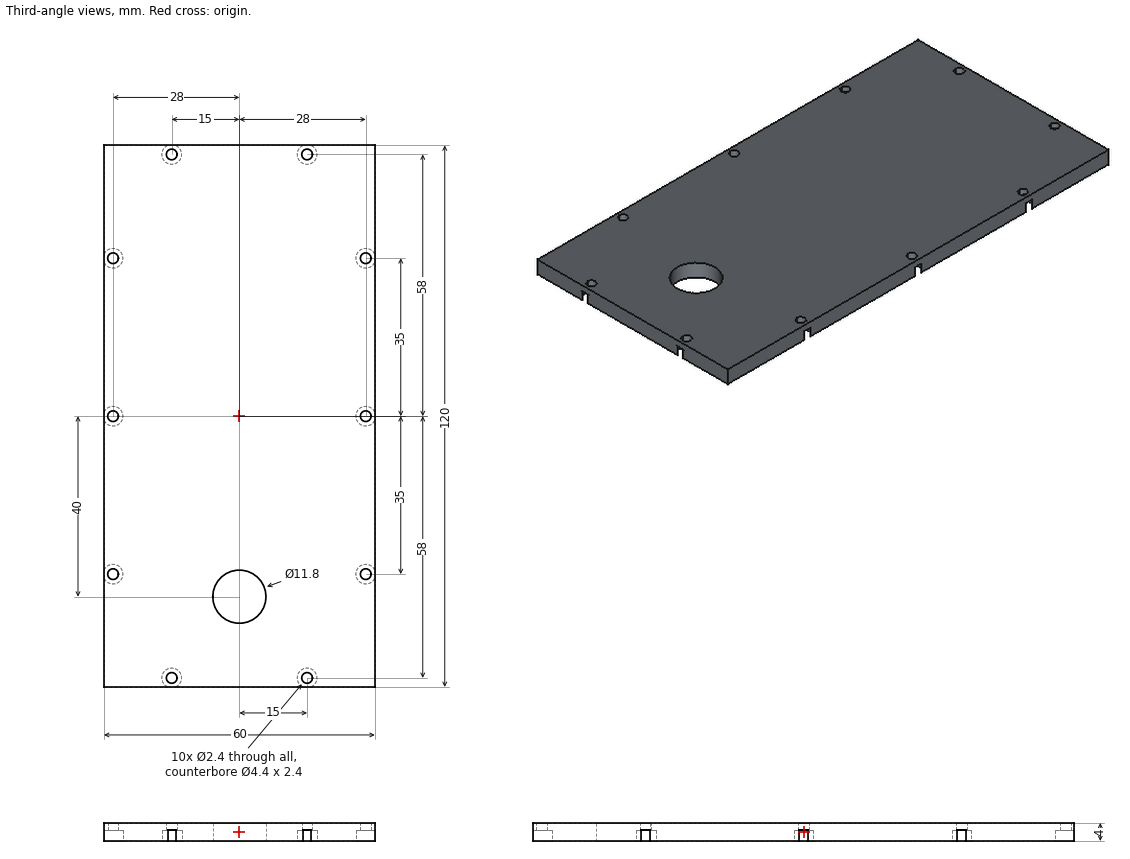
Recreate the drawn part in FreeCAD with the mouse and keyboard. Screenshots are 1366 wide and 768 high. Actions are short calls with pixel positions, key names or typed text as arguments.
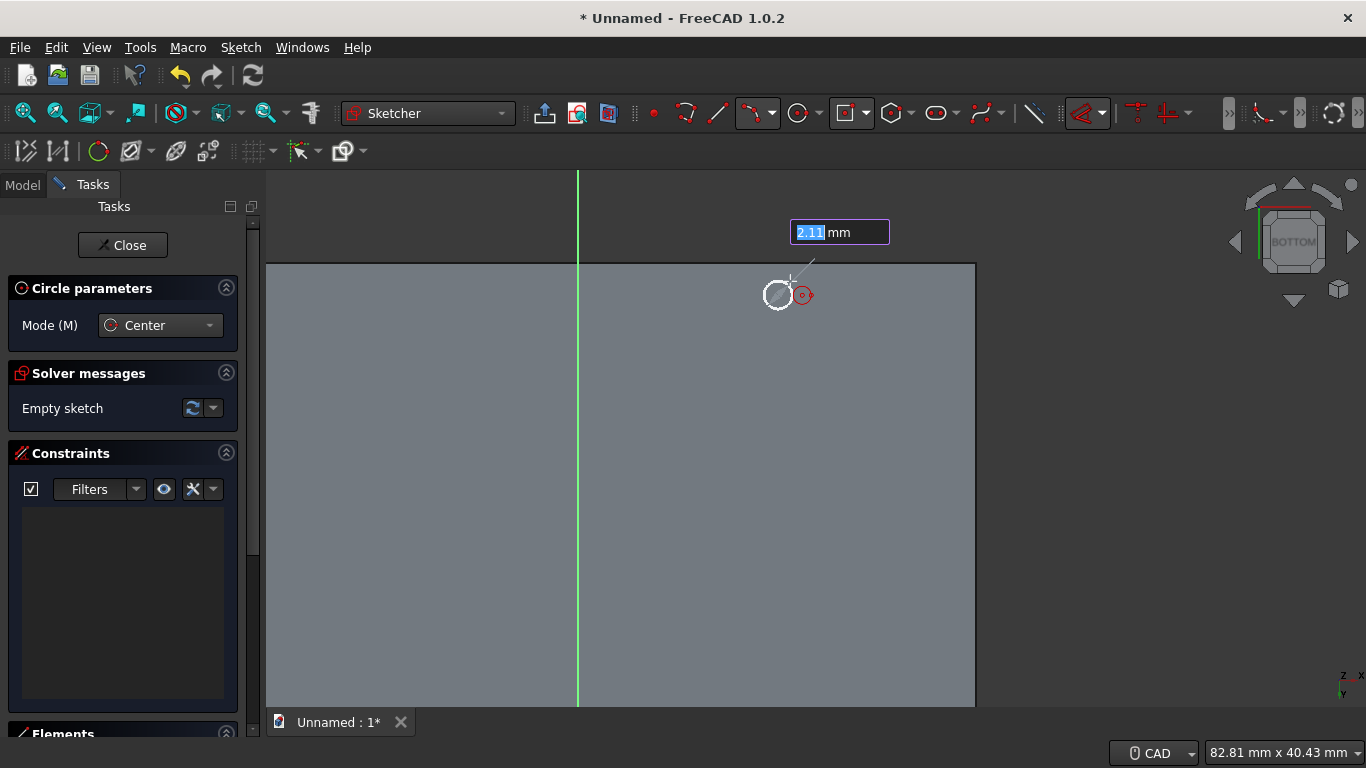
click(788, 279)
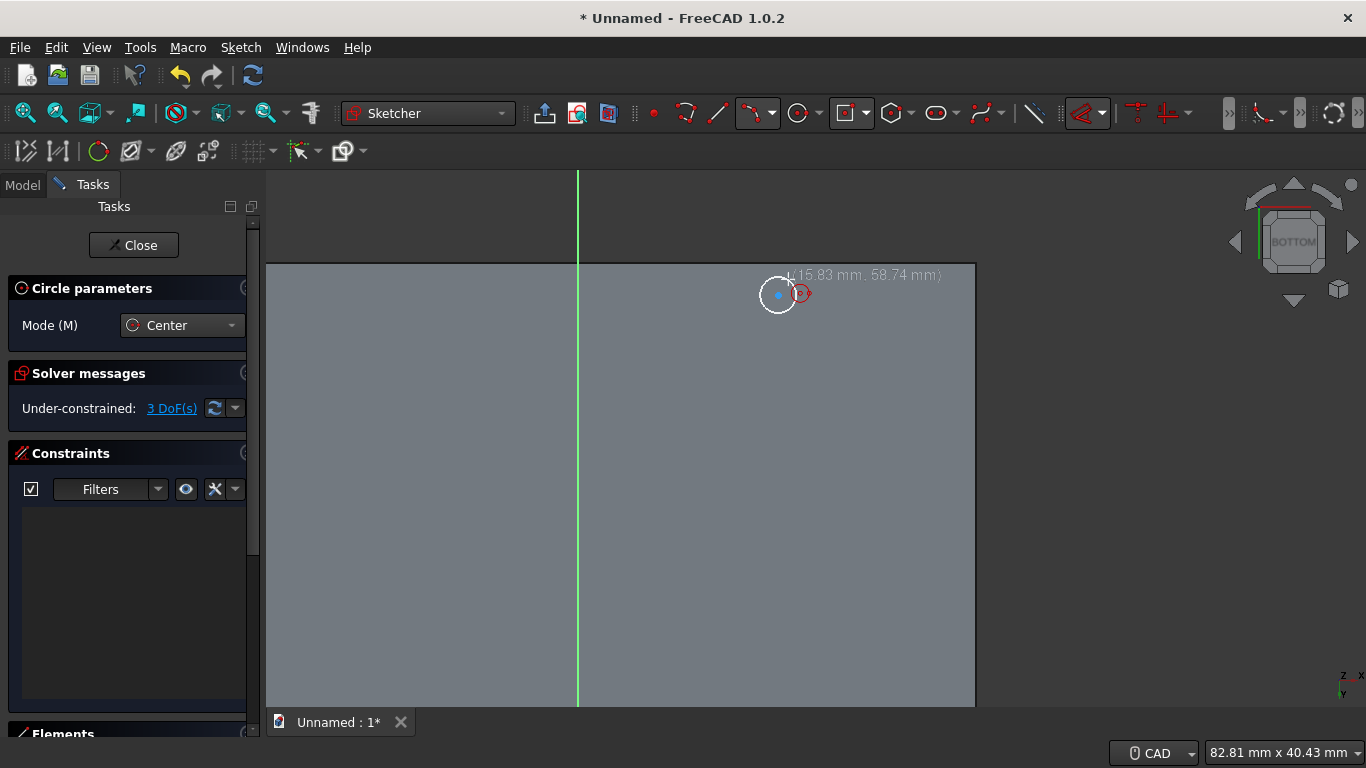
scroll(790, 281, down, 8)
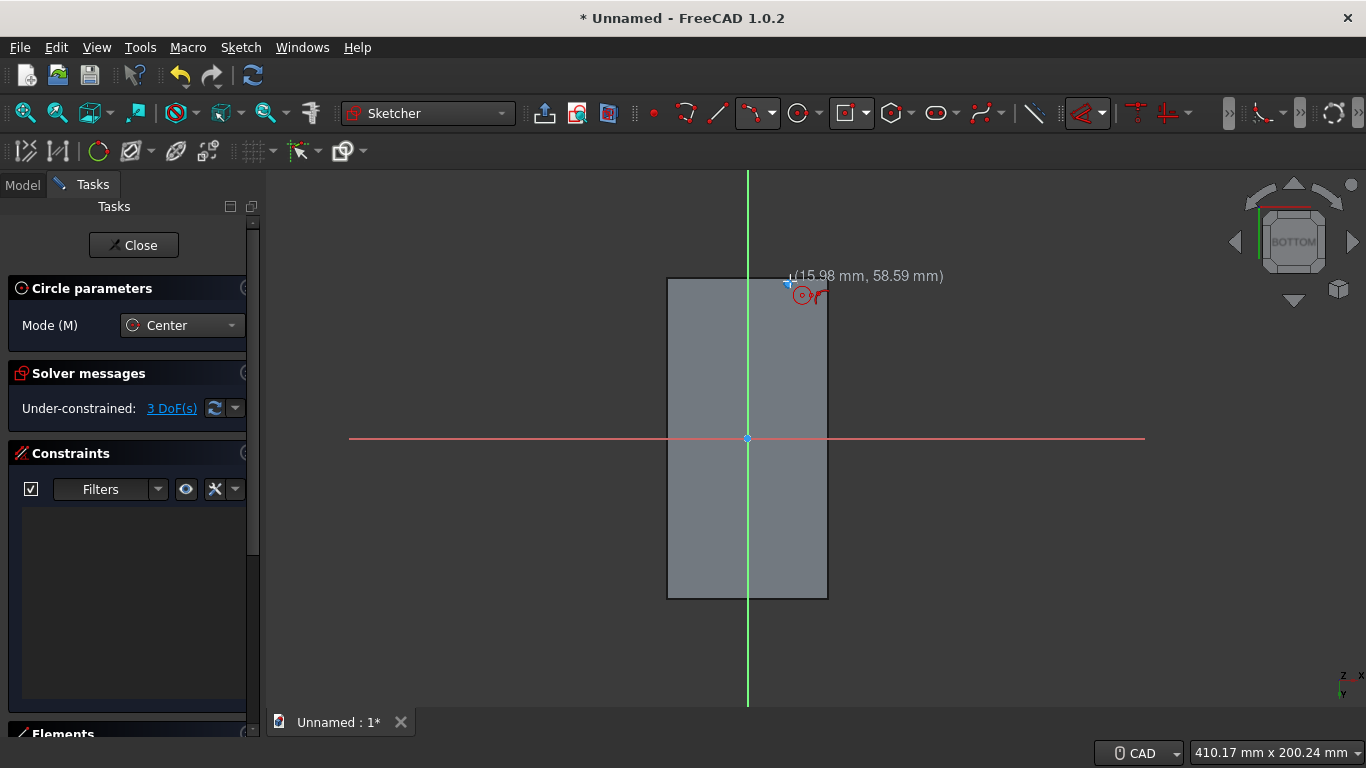
scroll(823, 438, up, 10)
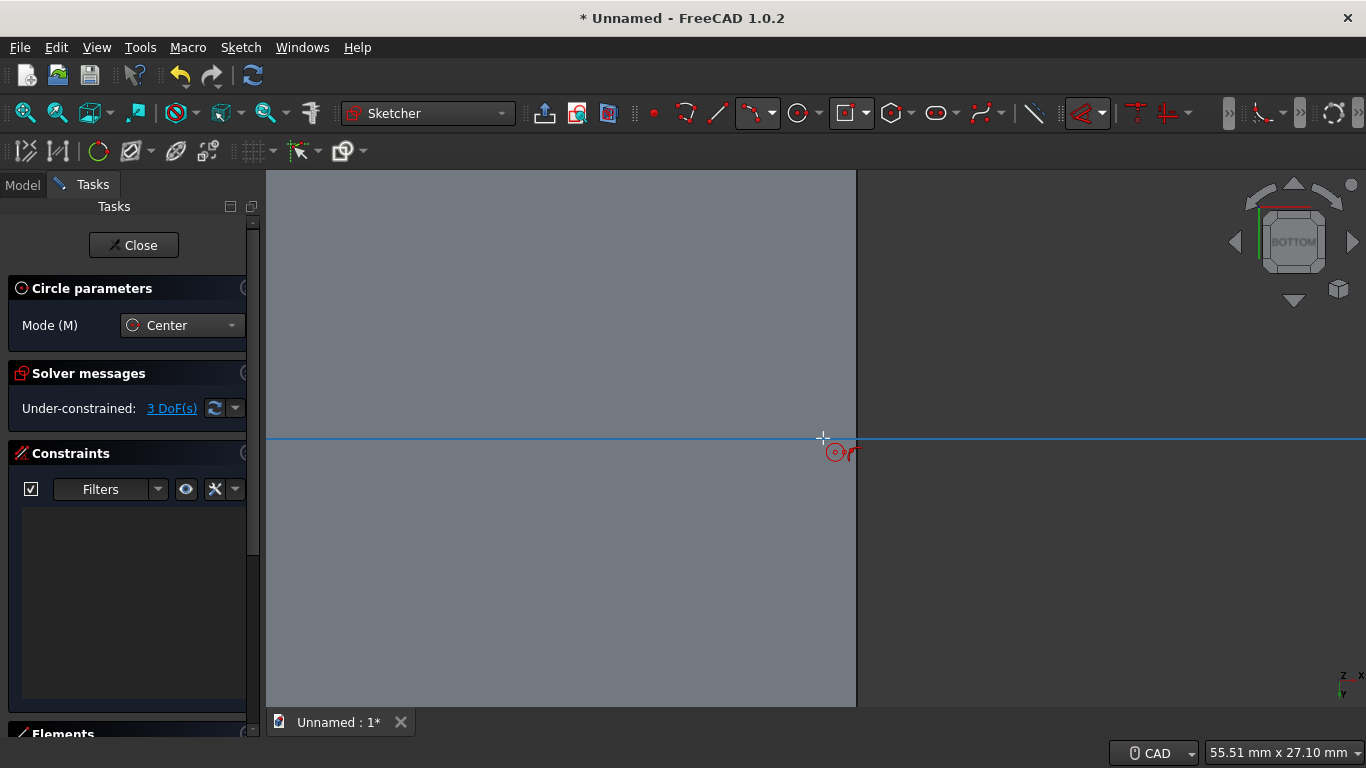
scroll(823, 439, down, 10)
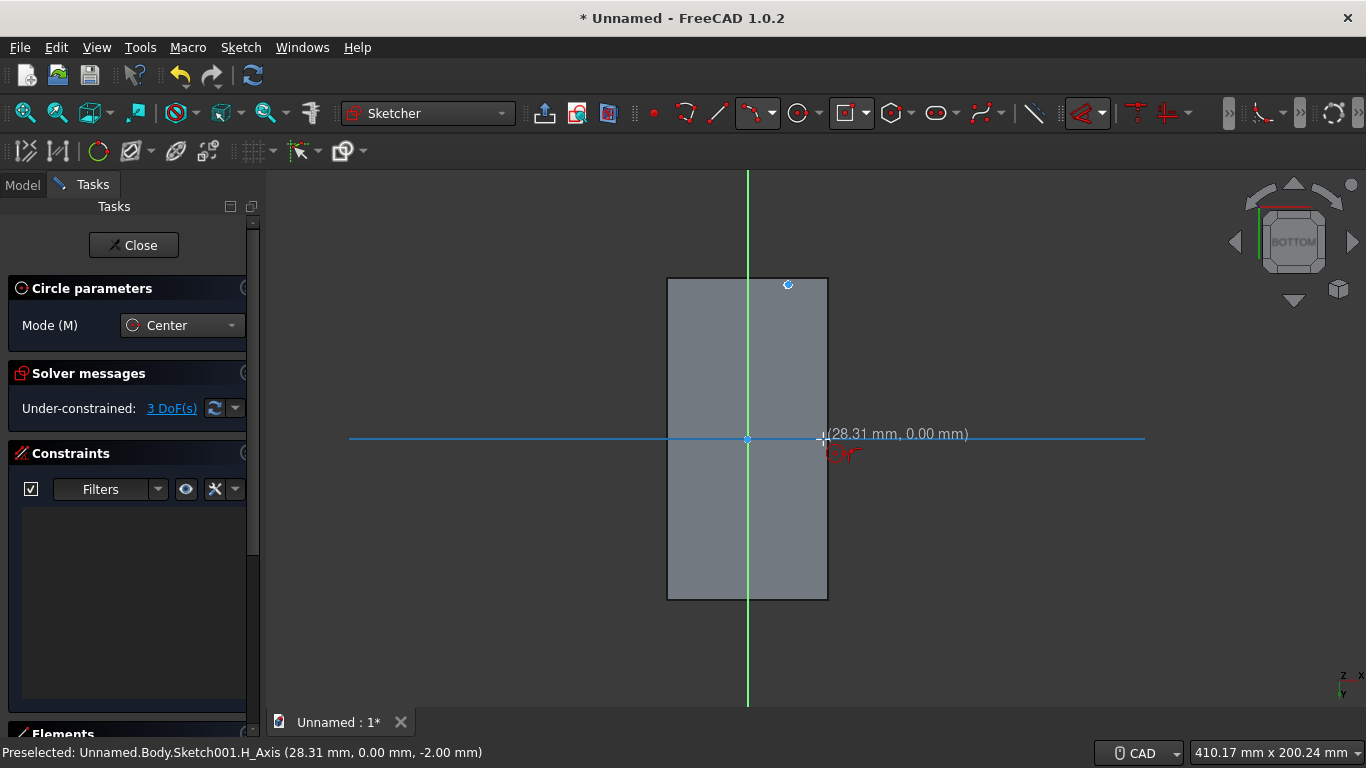
click(823, 439)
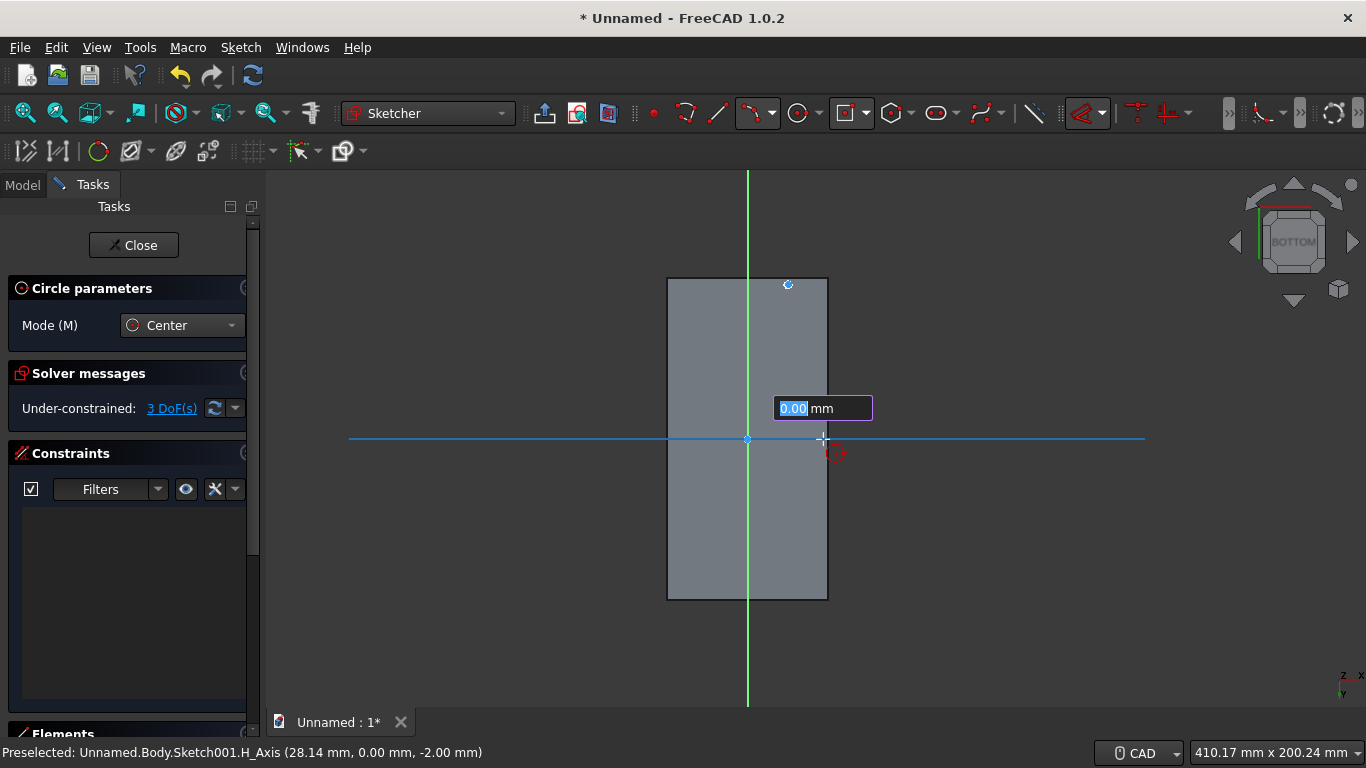
scroll(824, 436, up, 9)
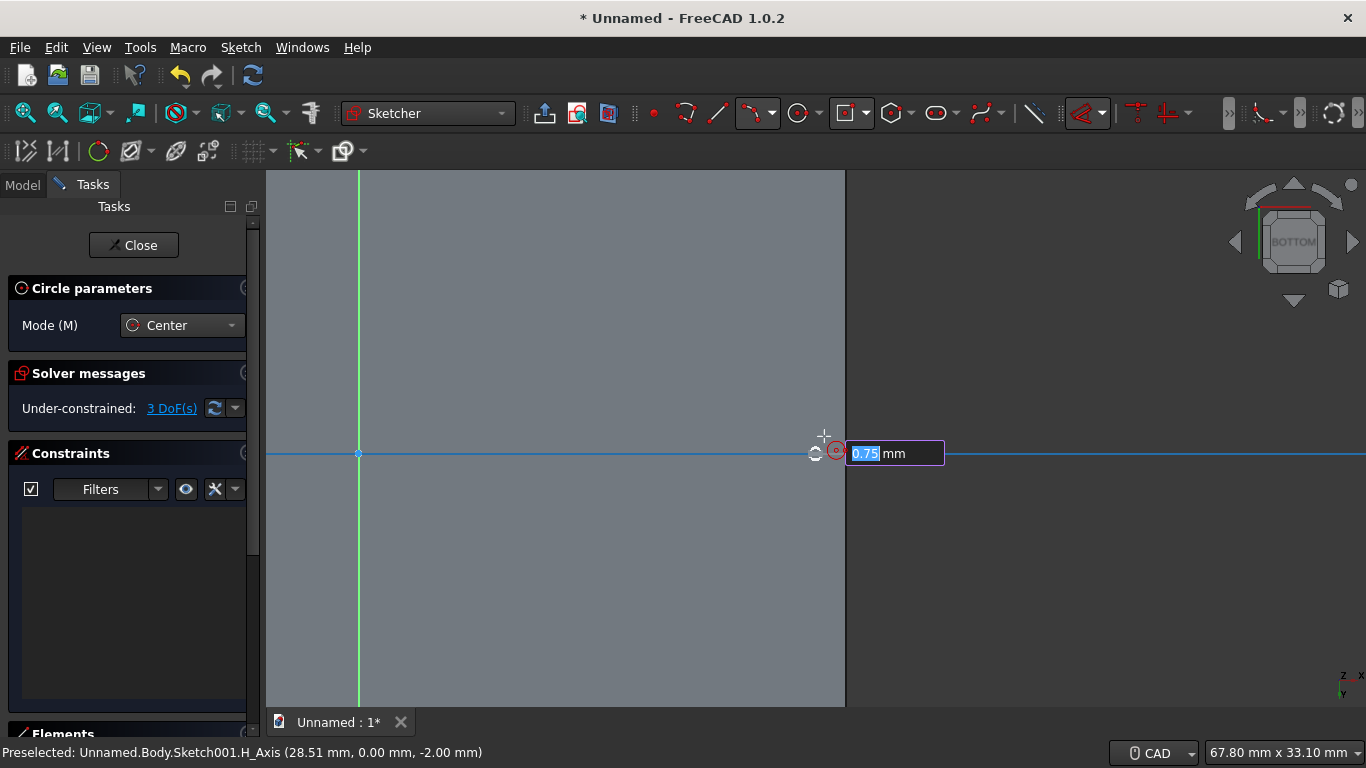
click(820, 436)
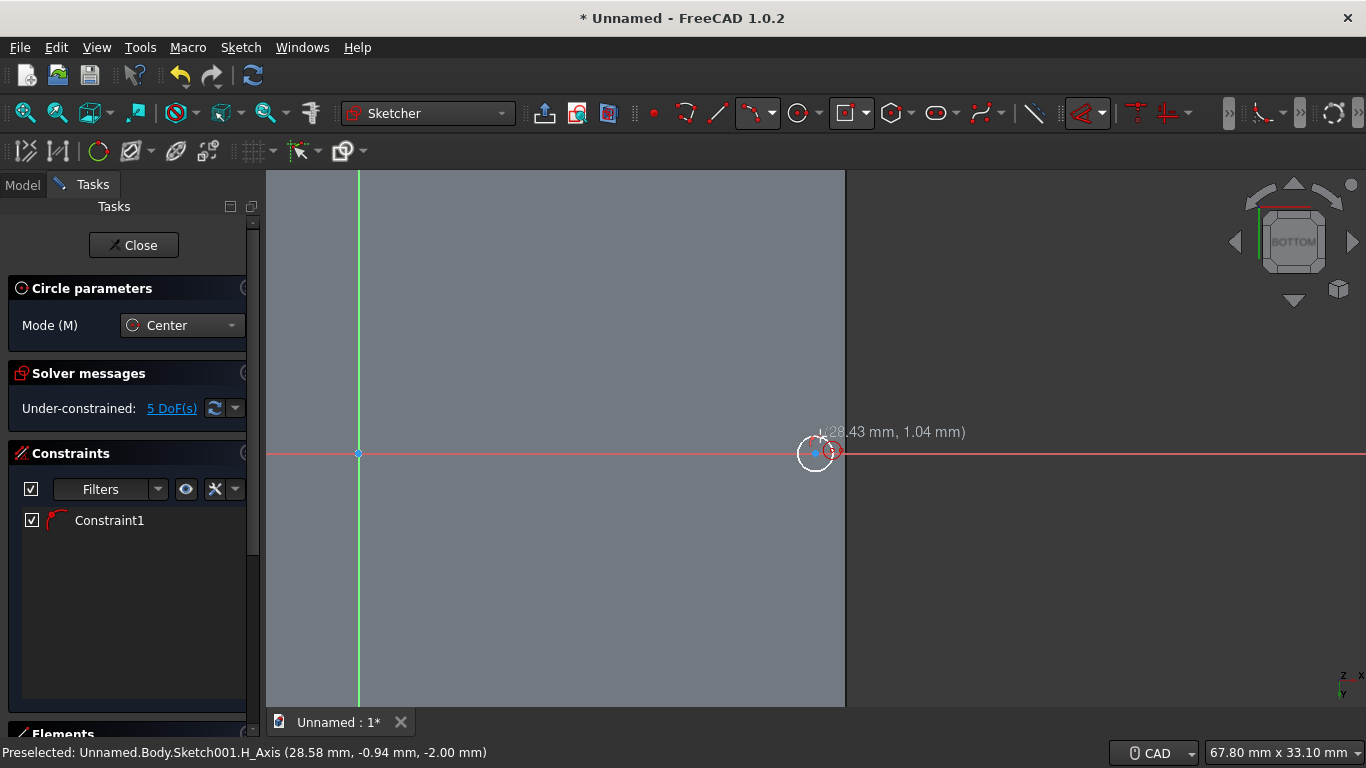
scroll(824, 435, down, 9)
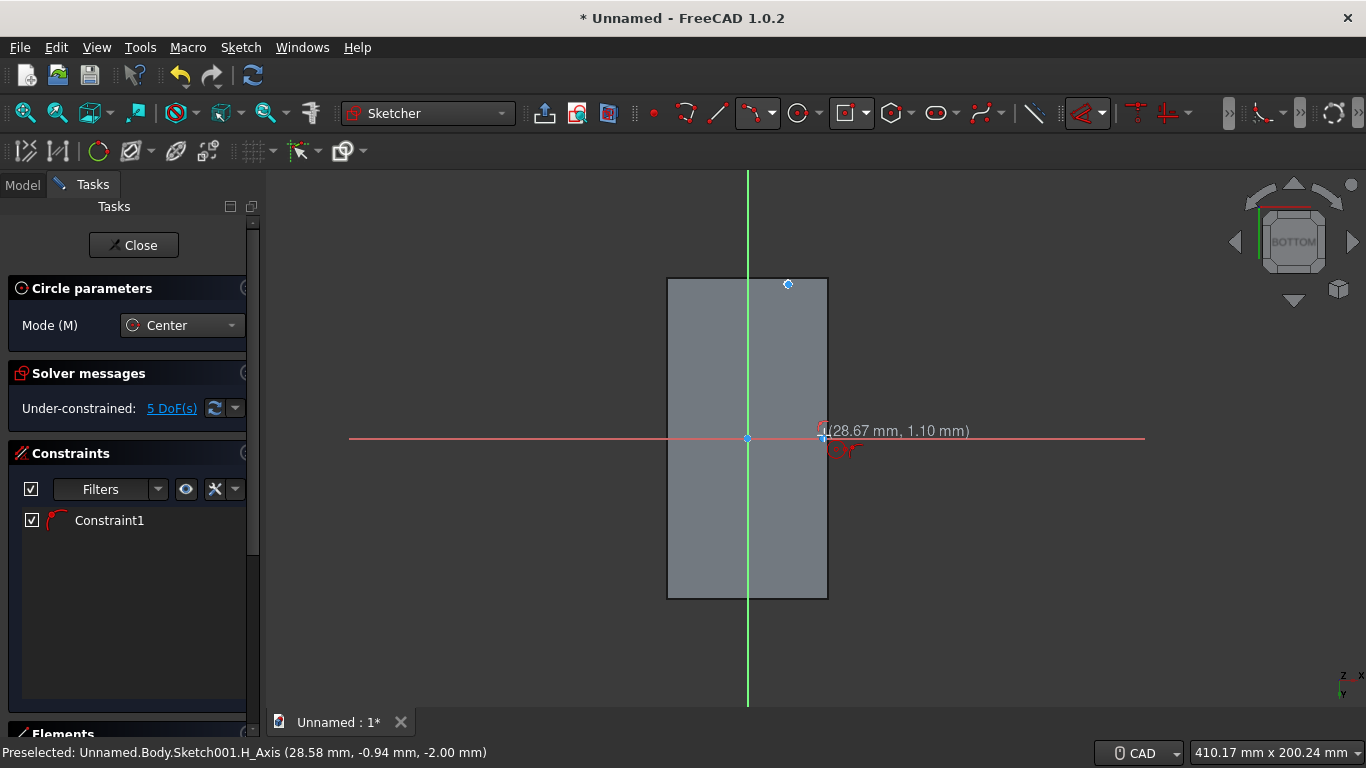
scroll(672, 439, up, 10)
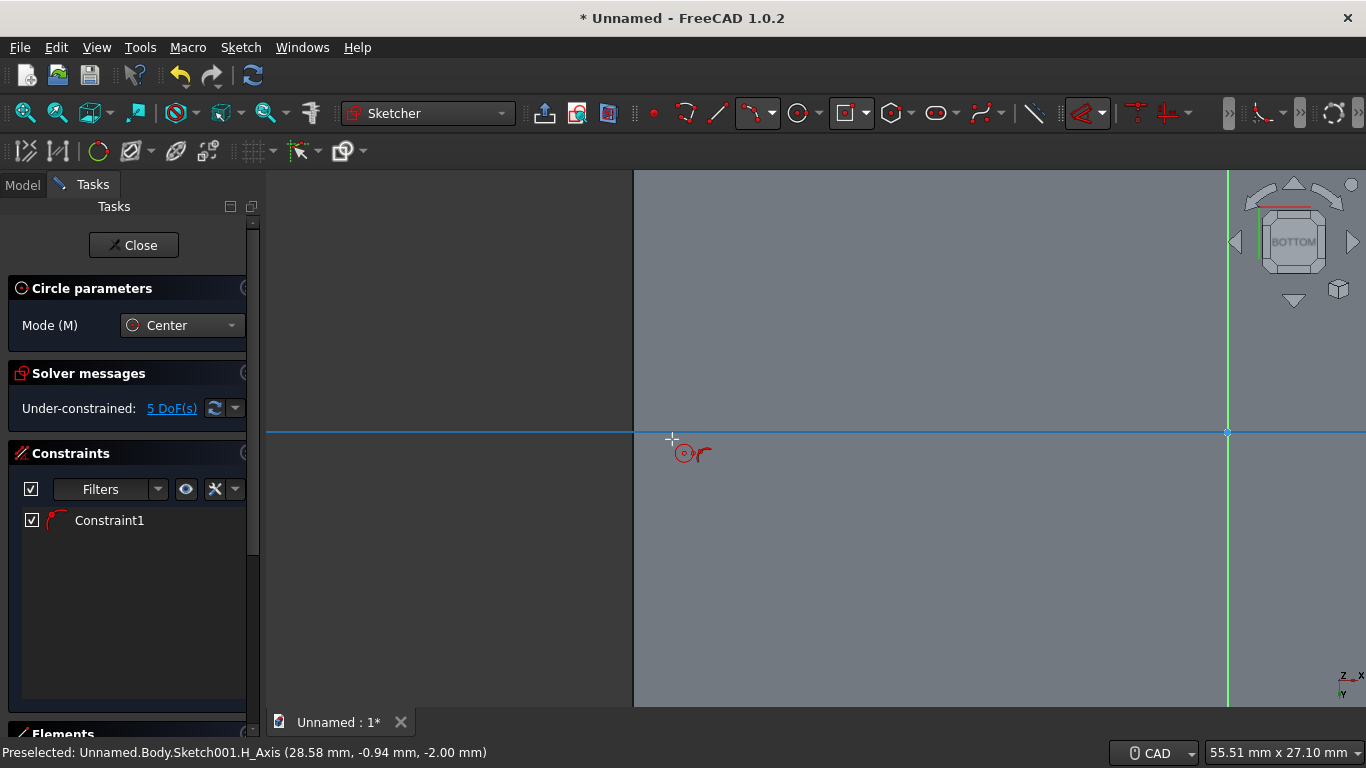
scroll(672, 439, down, 10)